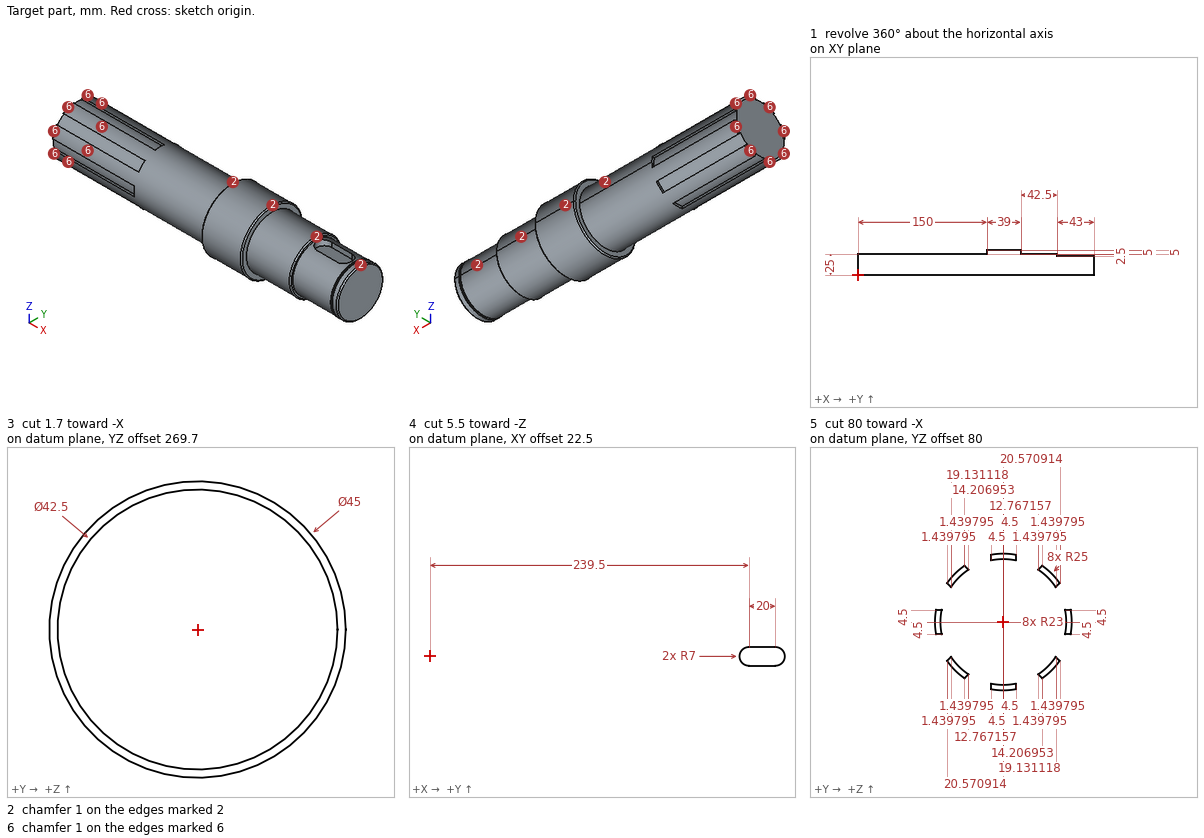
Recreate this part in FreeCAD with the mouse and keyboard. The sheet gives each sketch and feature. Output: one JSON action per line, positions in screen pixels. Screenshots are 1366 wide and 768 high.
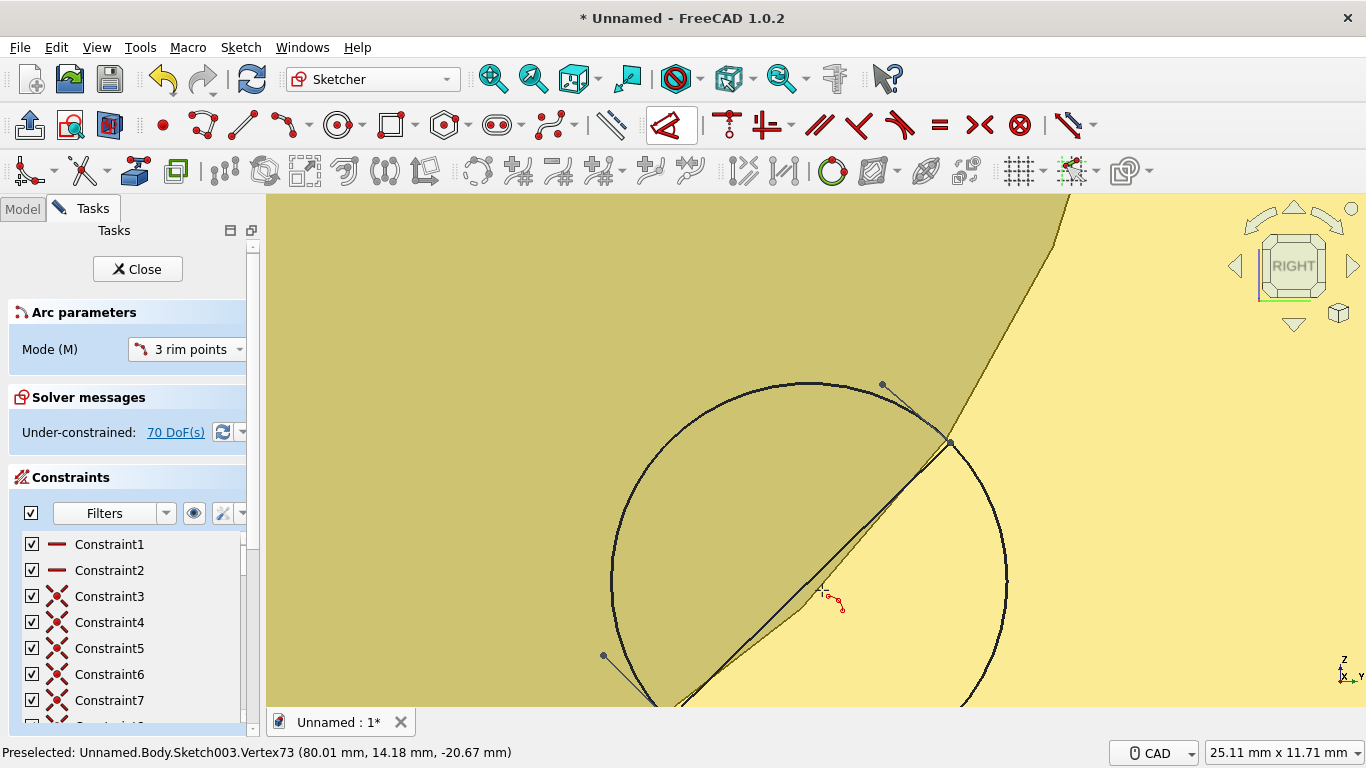
{"action": "left_click", "coordinate": [821, 589]}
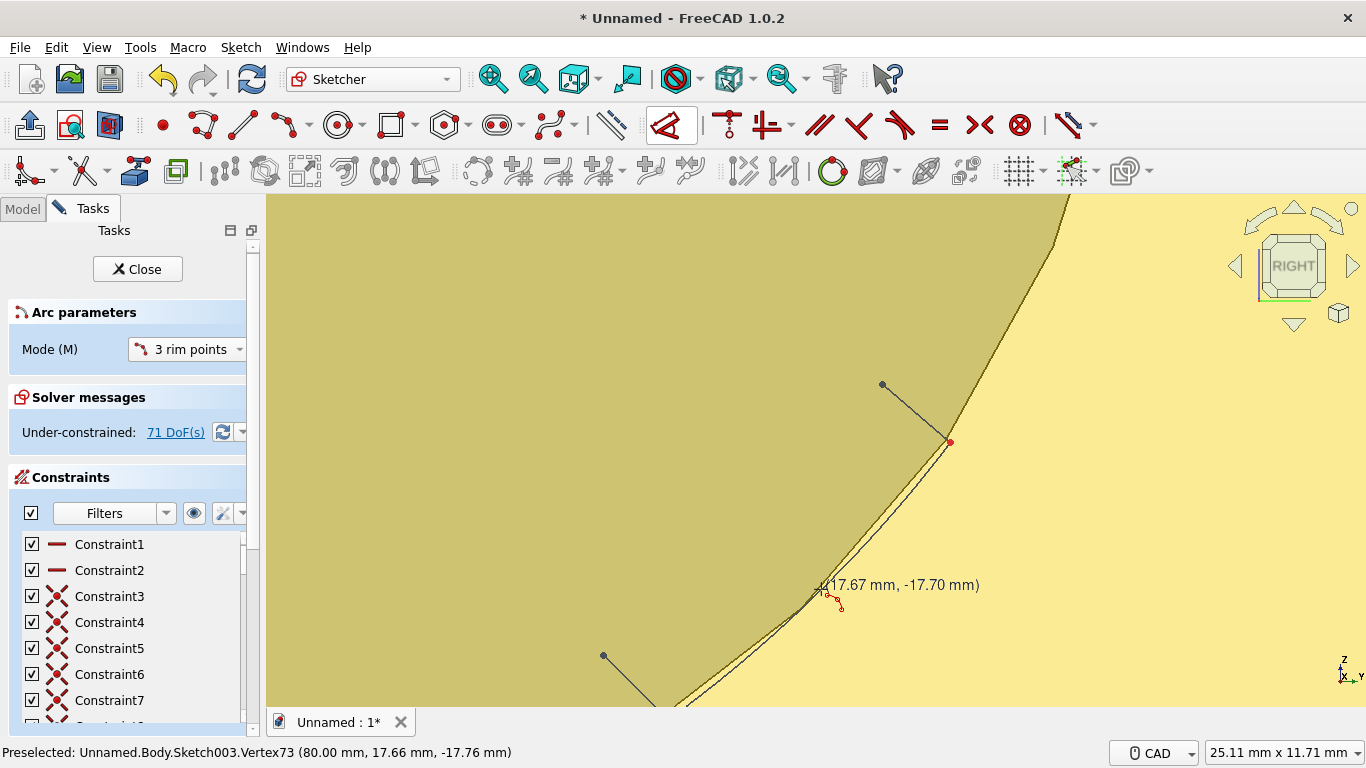
{"action": "left_click", "coordinate": [604, 656]}
{"action": "left_click", "coordinate": [883, 384]}
{"action": "left_click", "coordinate": [759, 527]}
{"action": "key", "text": "Escape"}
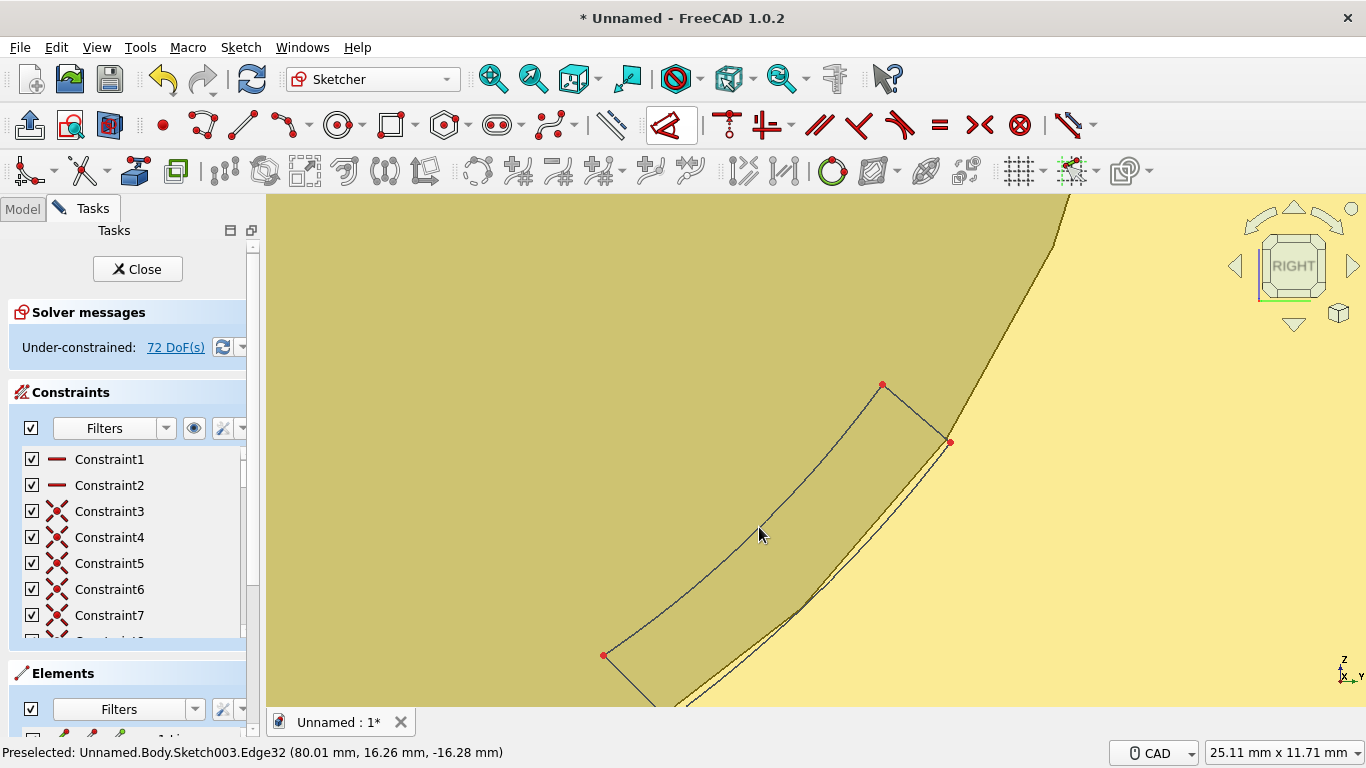
{"action": "scroll", "coordinate": [857, 550], "scroll_direction": "down", "scroll_amount": 10}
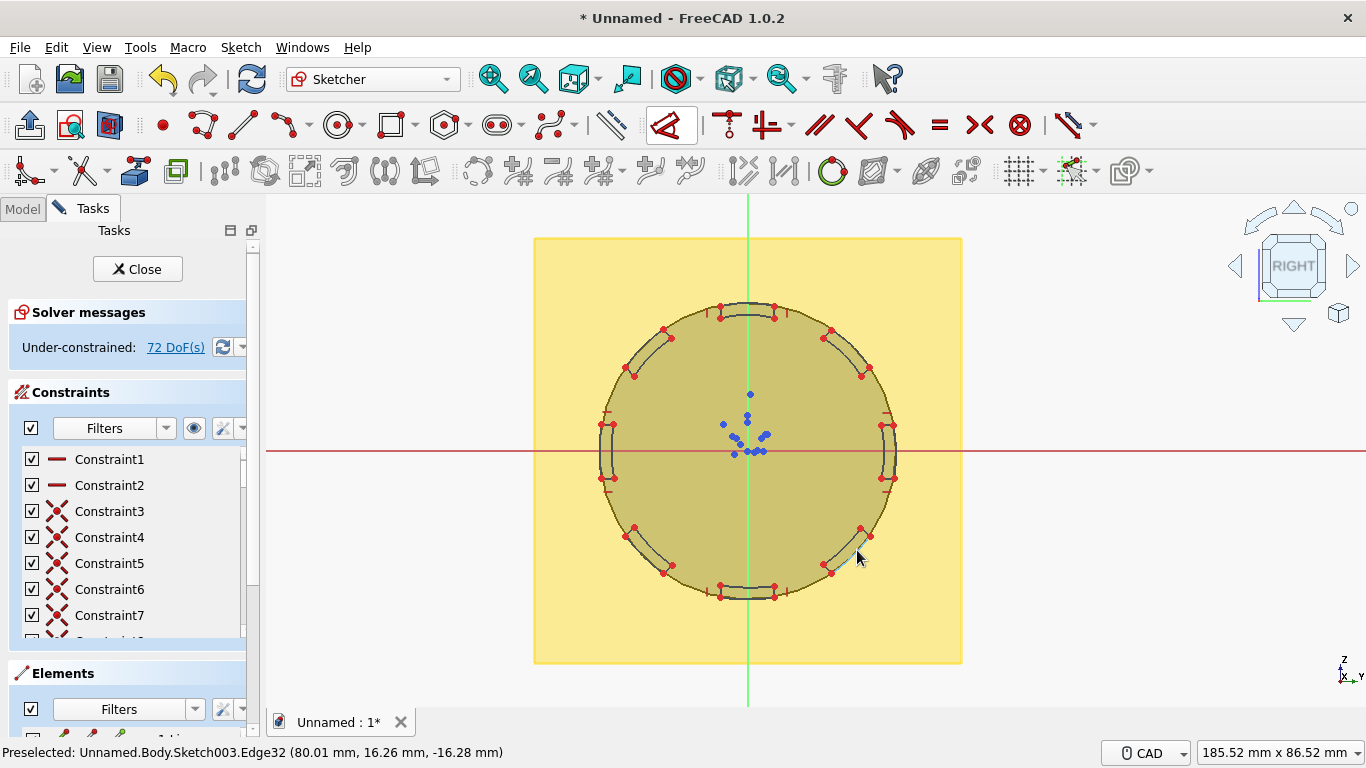
{"action": "left_click", "coordinate": [884, 463]}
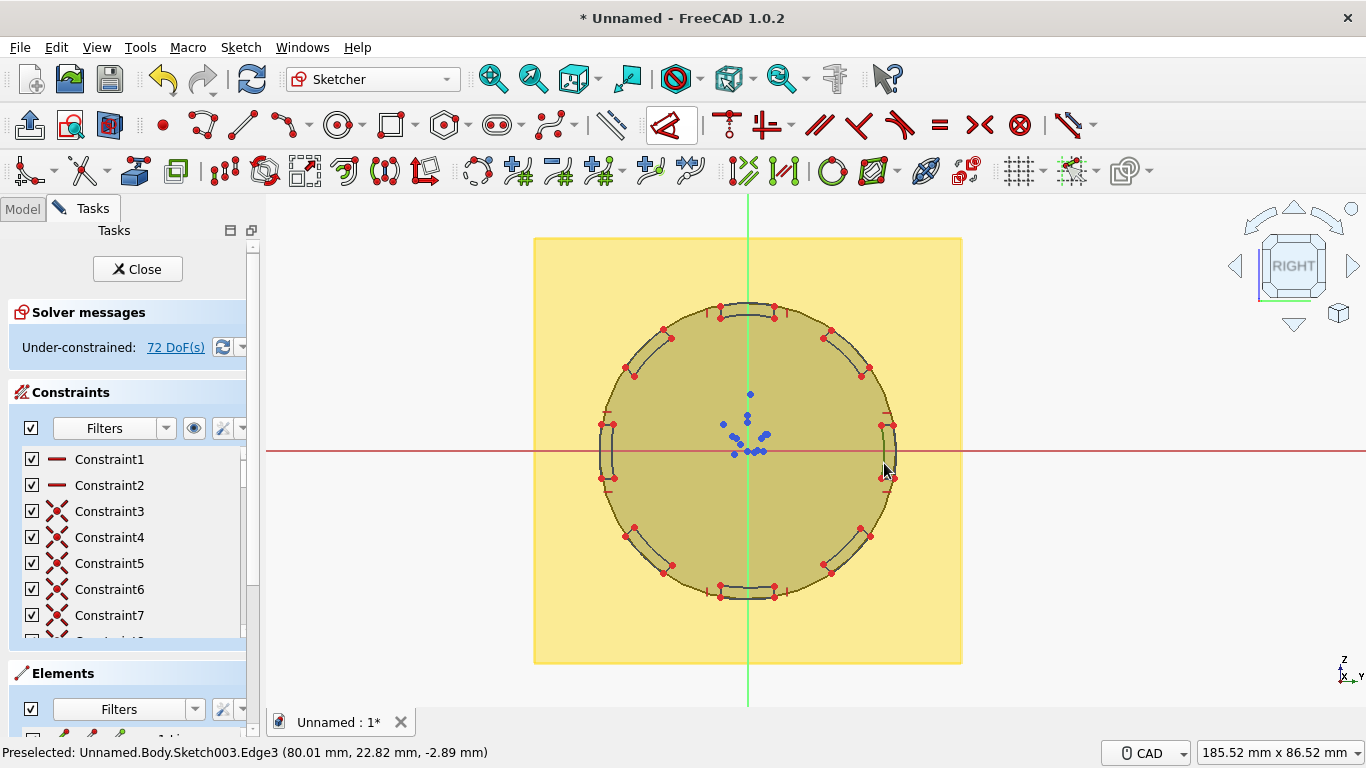
{"action": "left_click", "coordinate": [896, 463]}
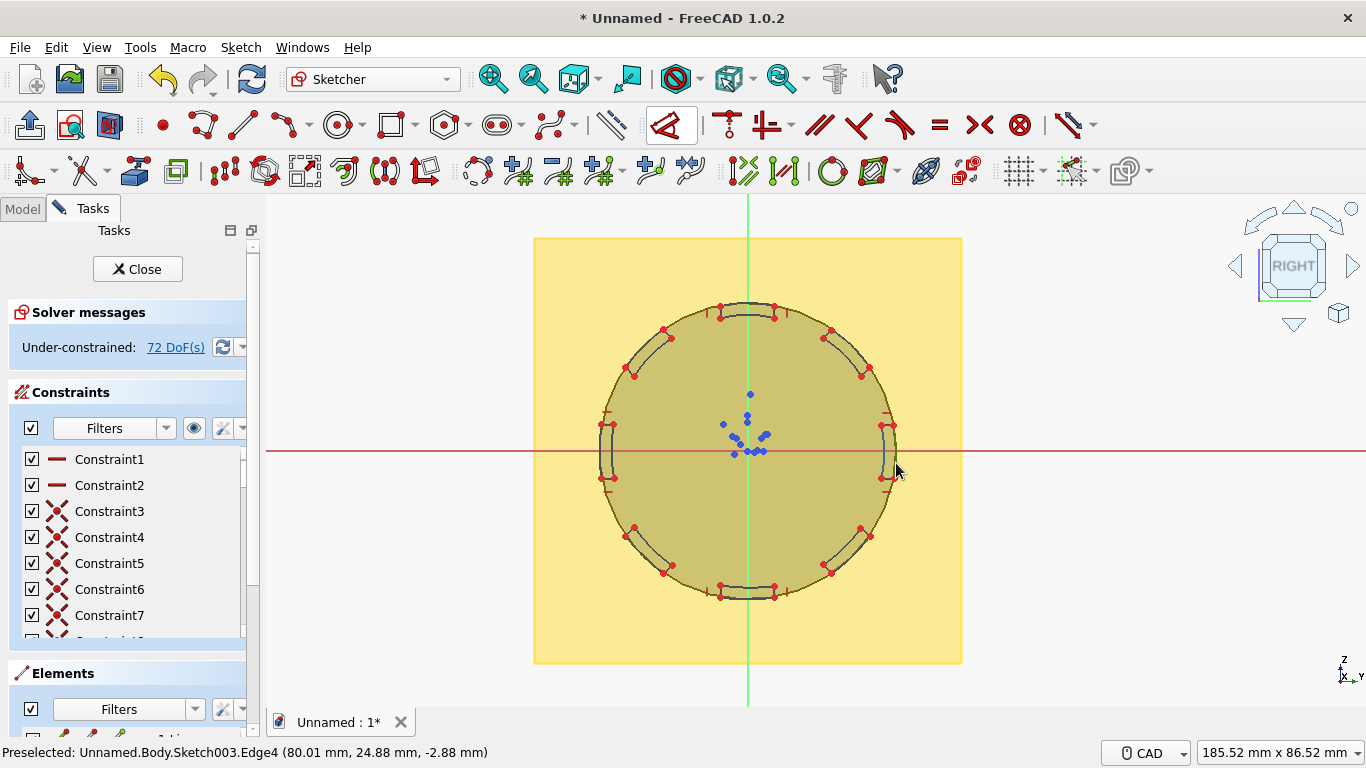
{"action": "key", "text": "c"}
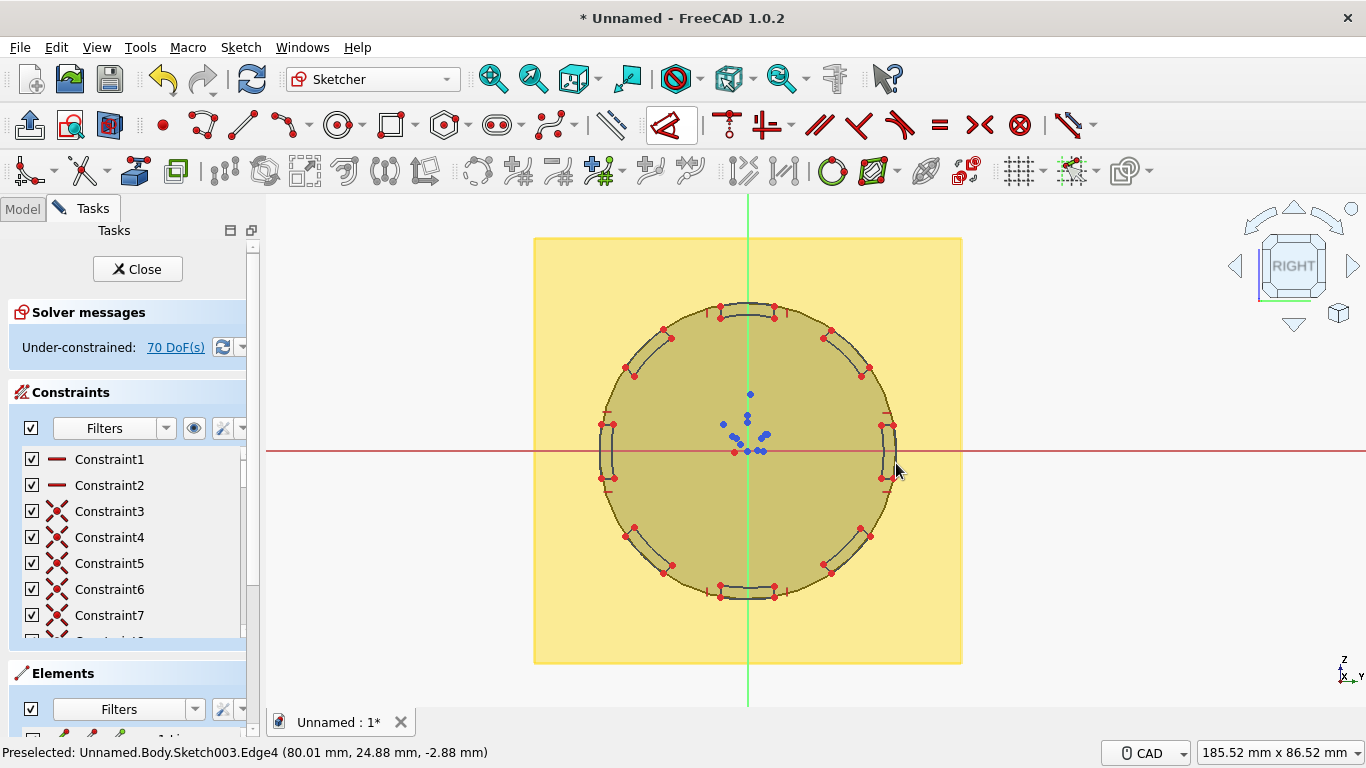
{"action": "left_click", "coordinate": [883, 463]}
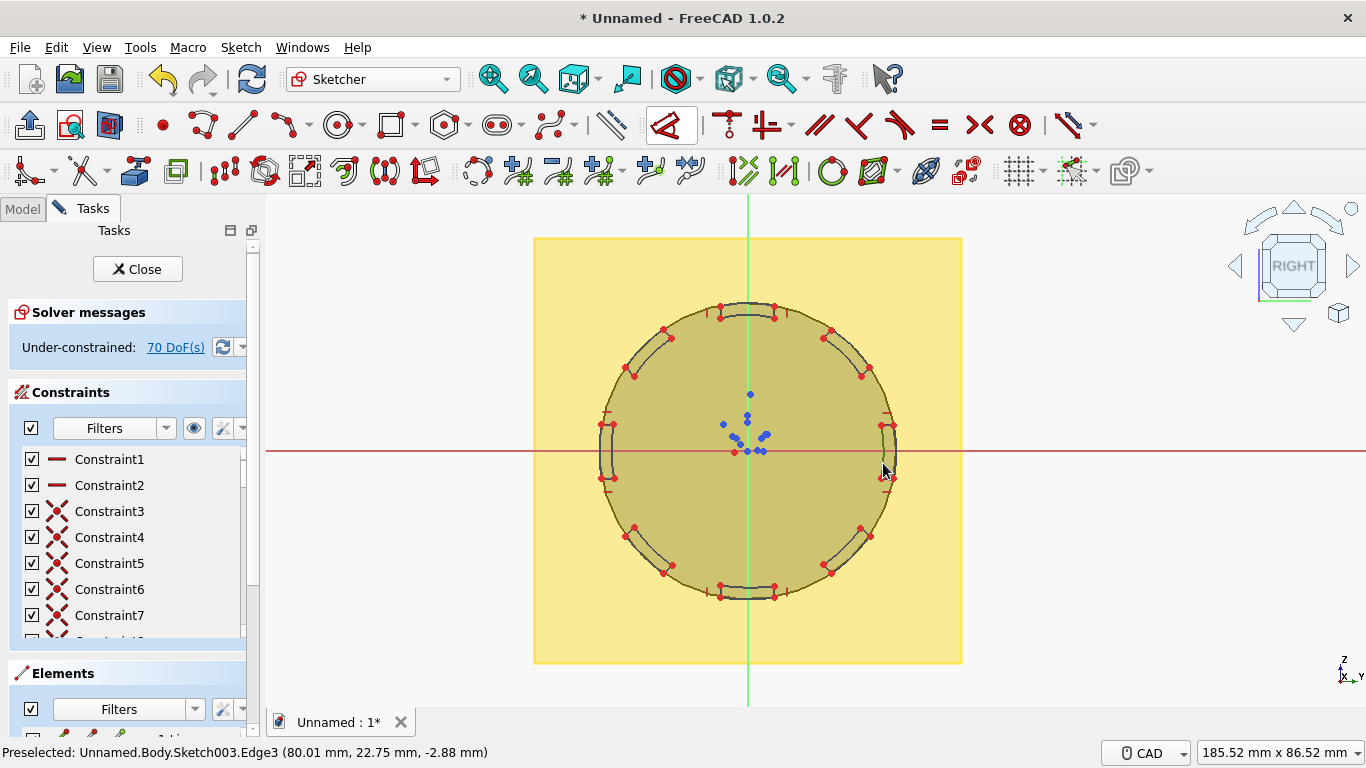
{"action": "left_click", "coordinate": [860, 355]}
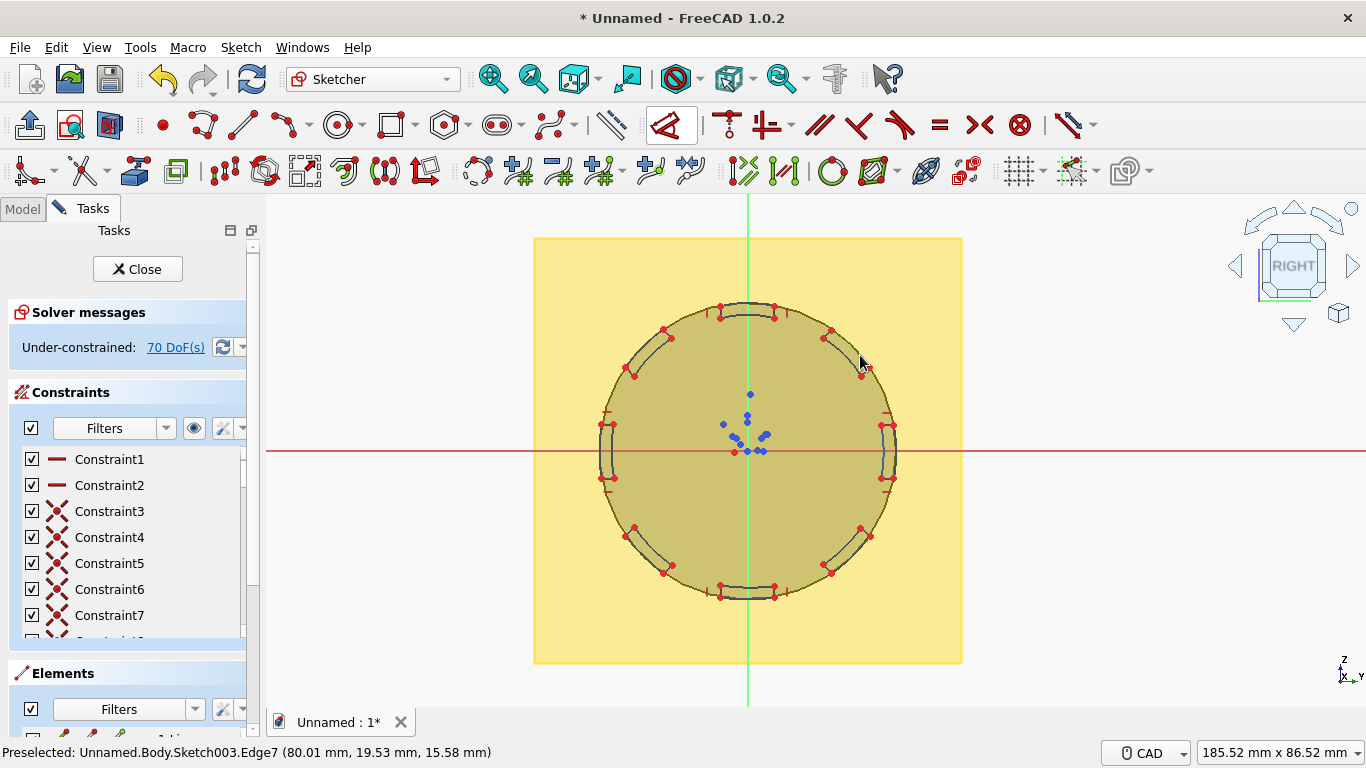
{"action": "left_click", "coordinate": [728, 126]}